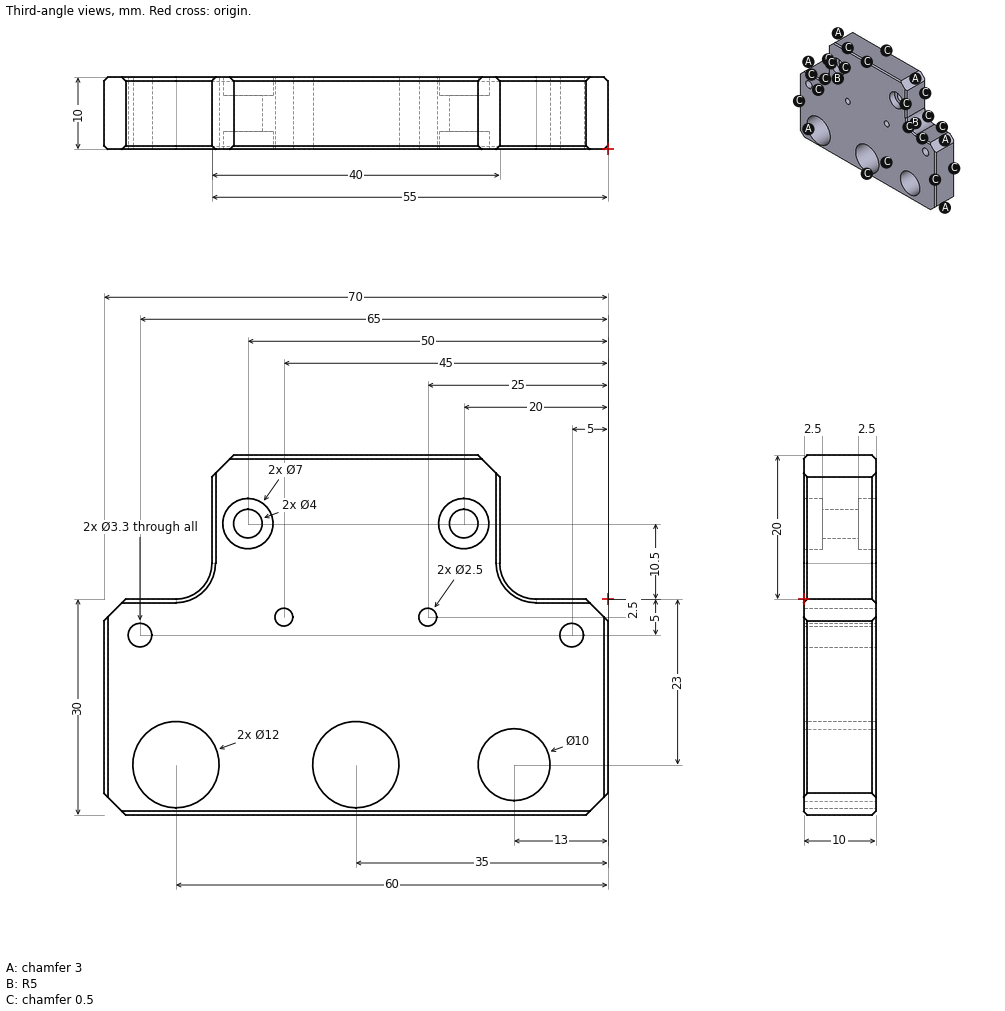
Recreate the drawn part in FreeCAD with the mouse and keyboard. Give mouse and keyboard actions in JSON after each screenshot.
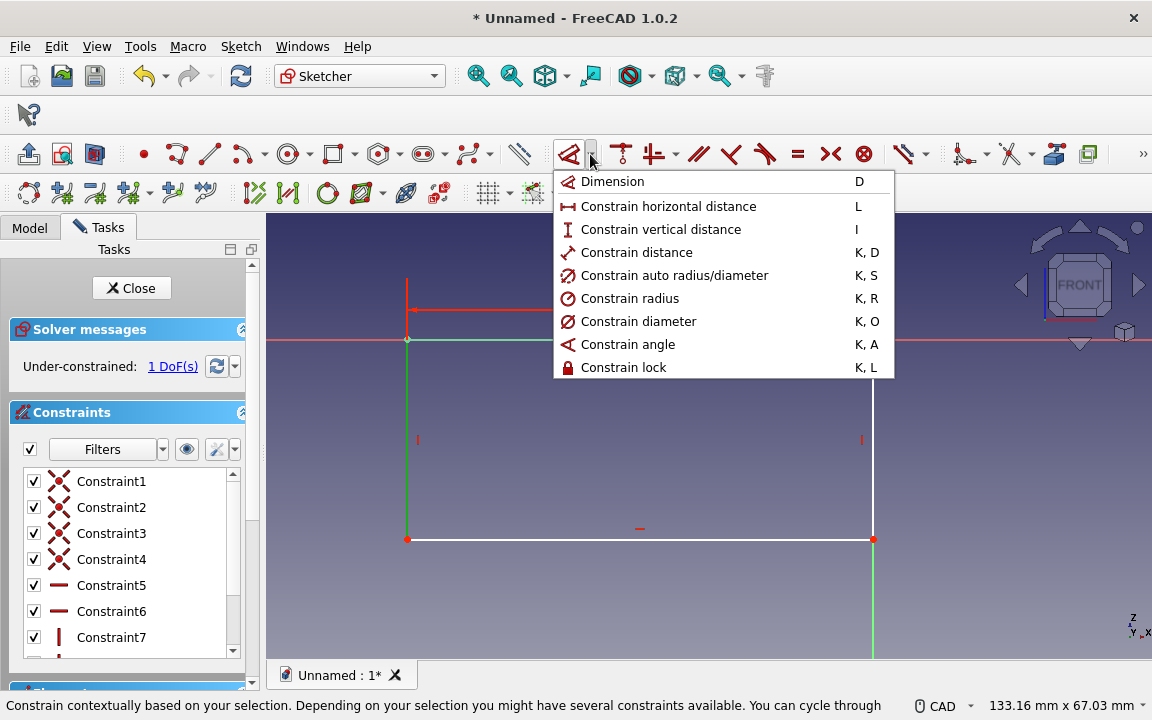
{"action": "left_click", "coordinate": [724, 230]}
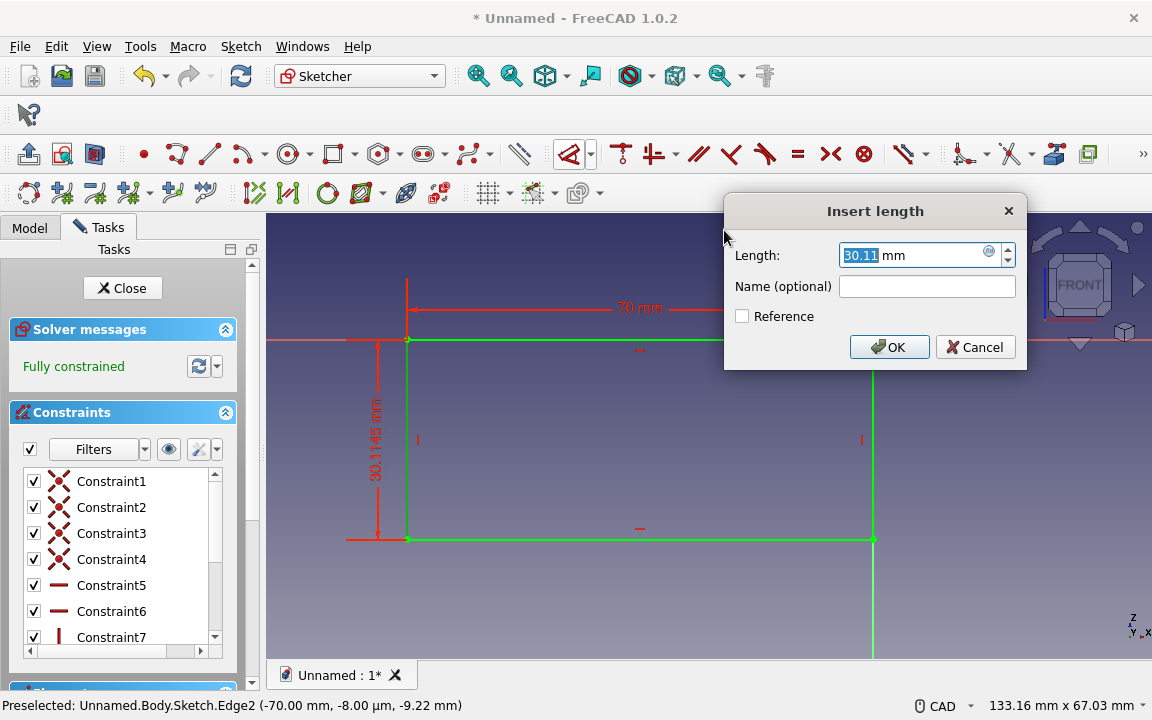
{"action": "type", "text": "30"}
{"action": "key", "text": "Return"}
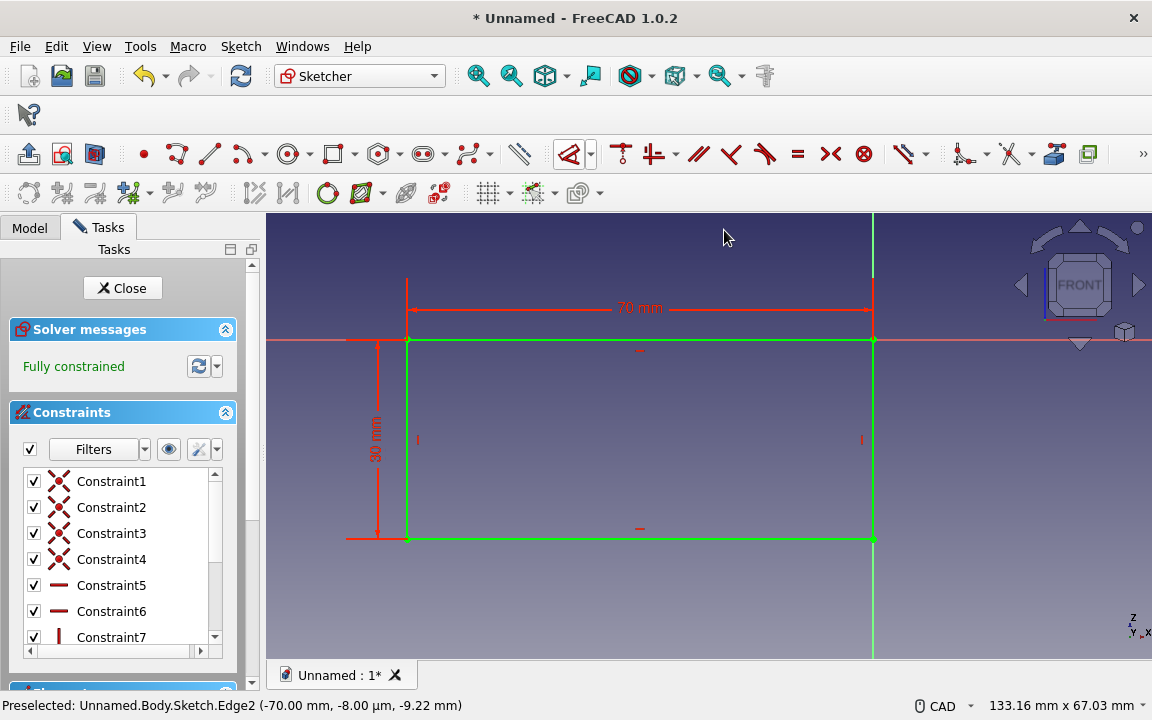
{"action": "left_click", "coordinate": [123, 288]}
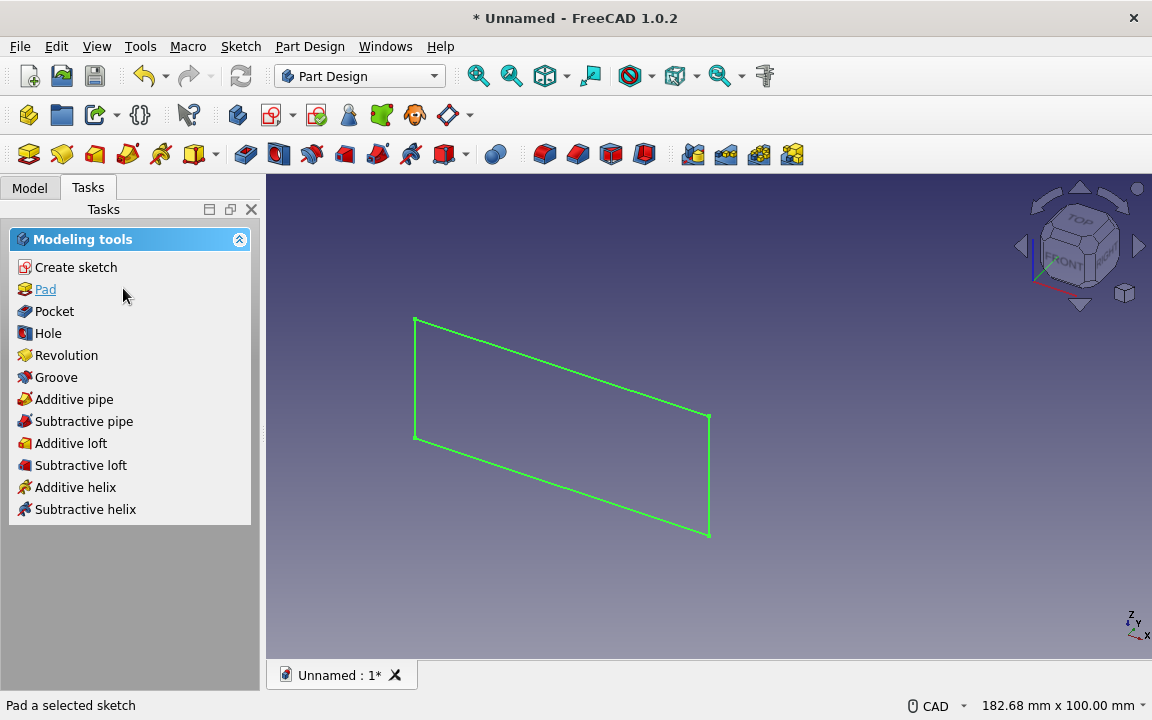
{"action": "left_click", "coordinate": [29, 154]}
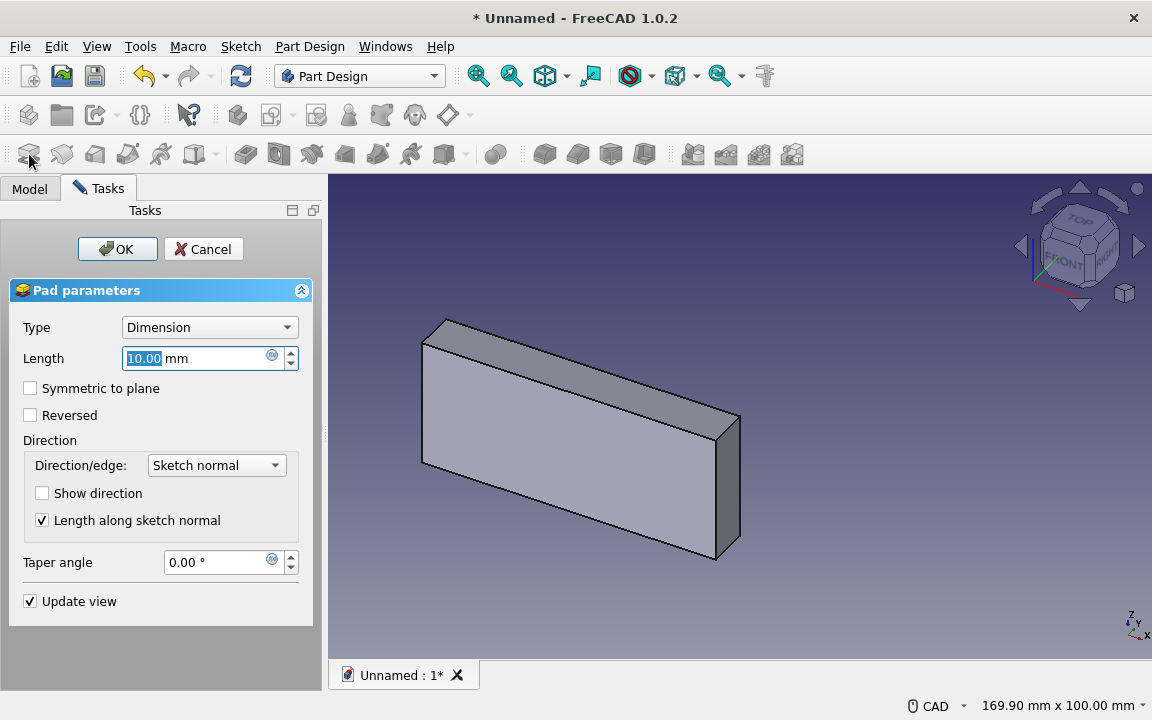
{"action": "type", "text": "10"}
{"action": "key", "text": "Tab"}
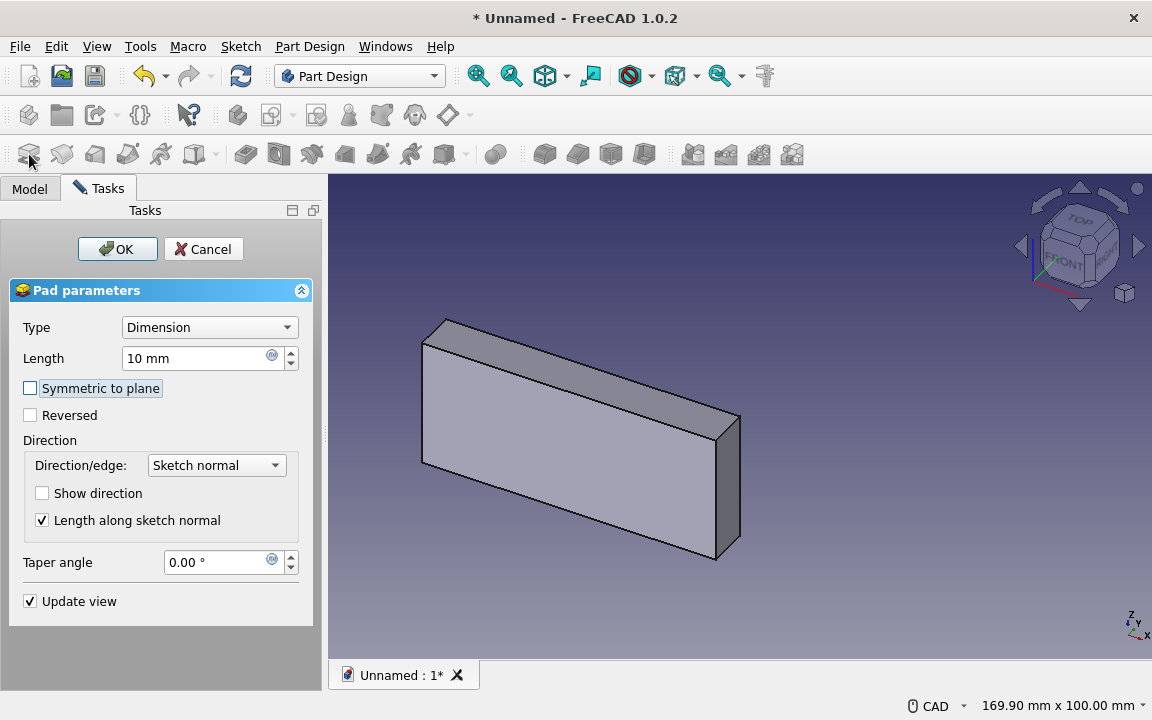
{"action": "left_click", "coordinate": [31, 415]}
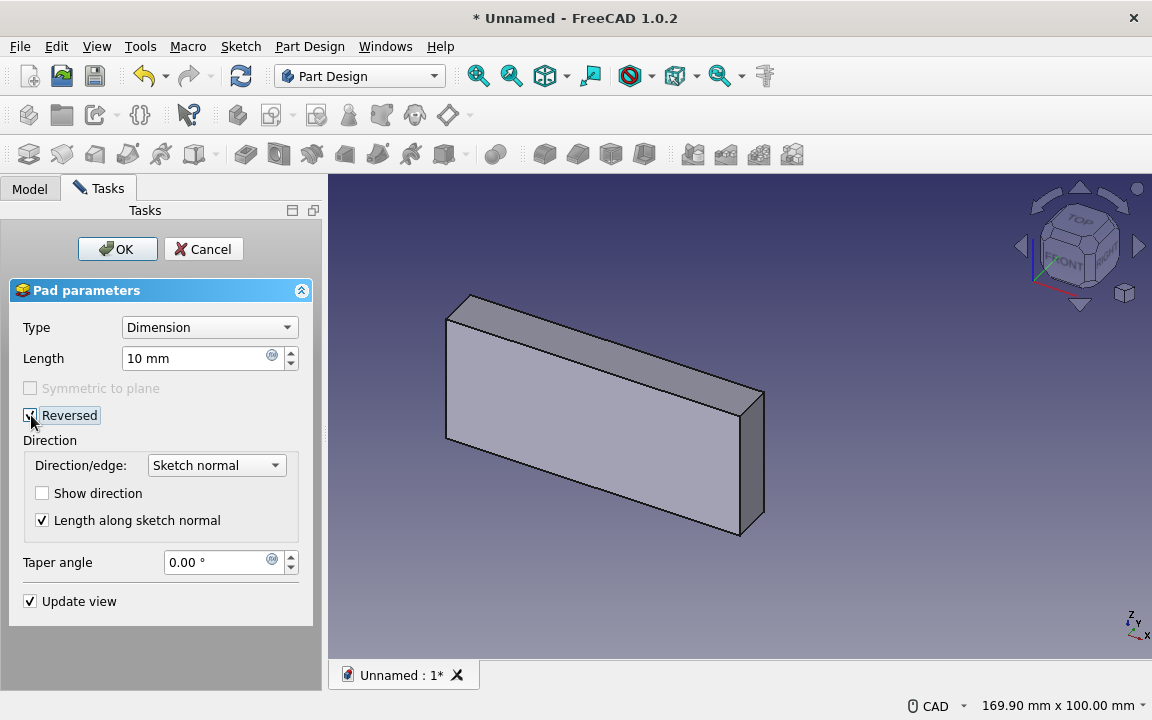
{"action": "left_click", "coordinate": [118, 249]}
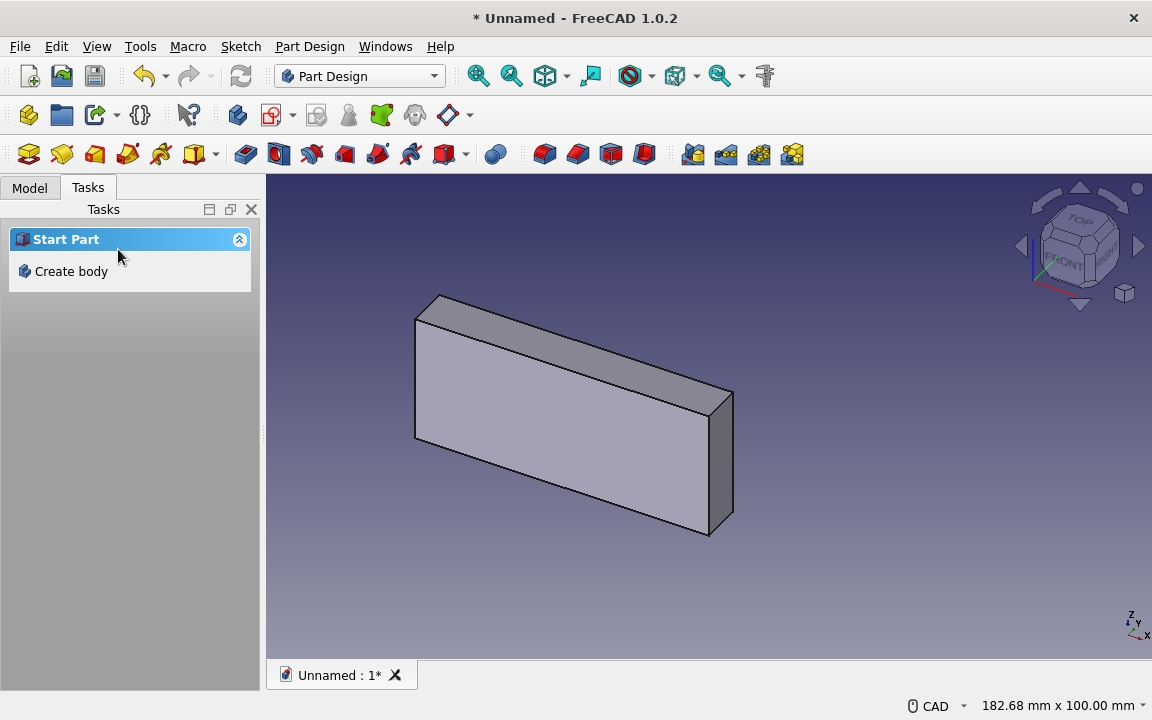
{"action": "left_click", "coordinate": [646, 454]}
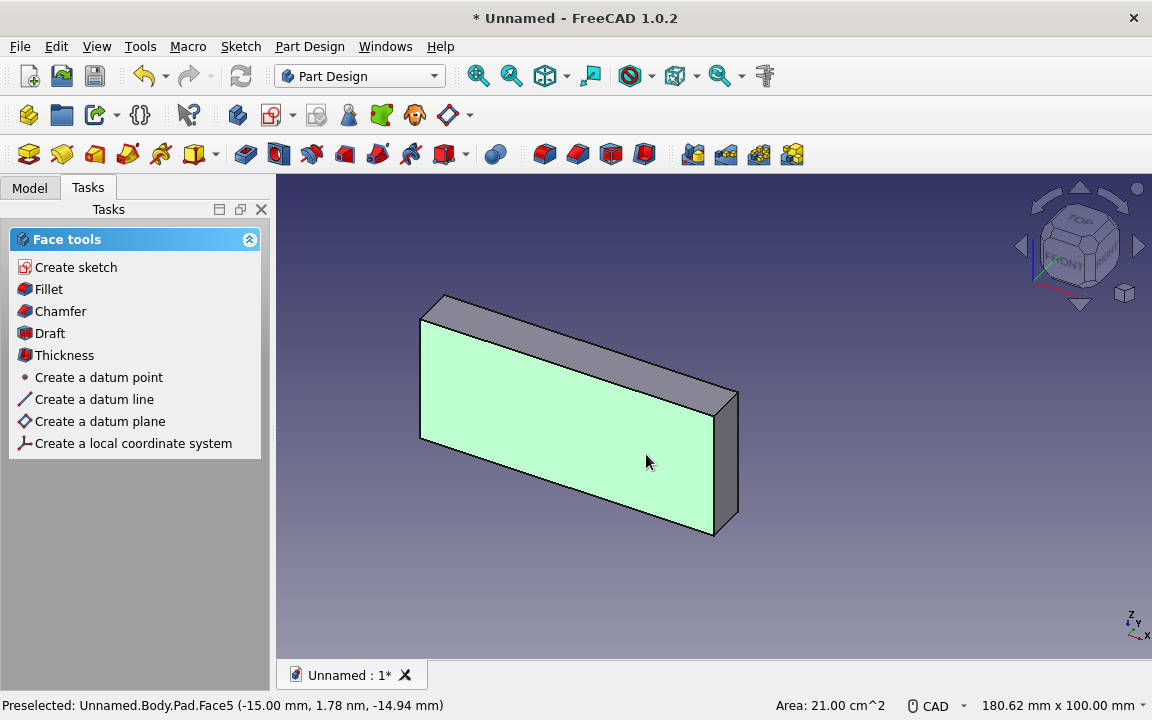
{"action": "left_click", "coordinate": [270, 116]}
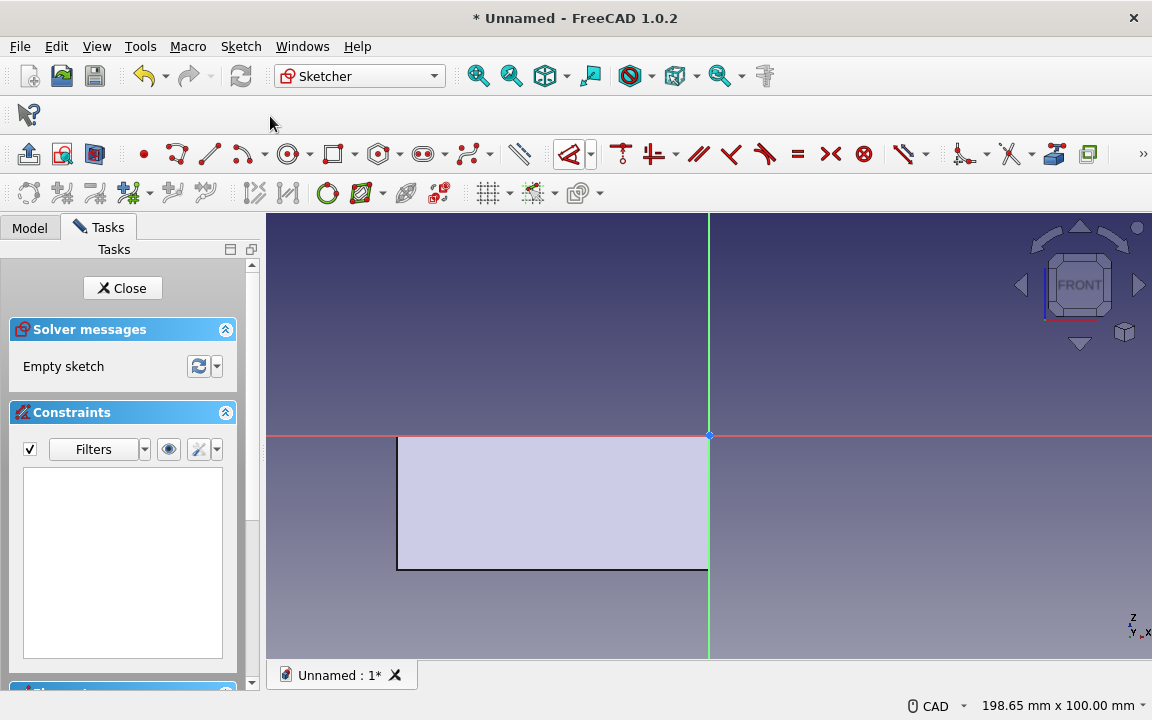
{"action": "scroll", "coordinate": [653, 559], "scroll_direction": "up", "scroll_amount": 9}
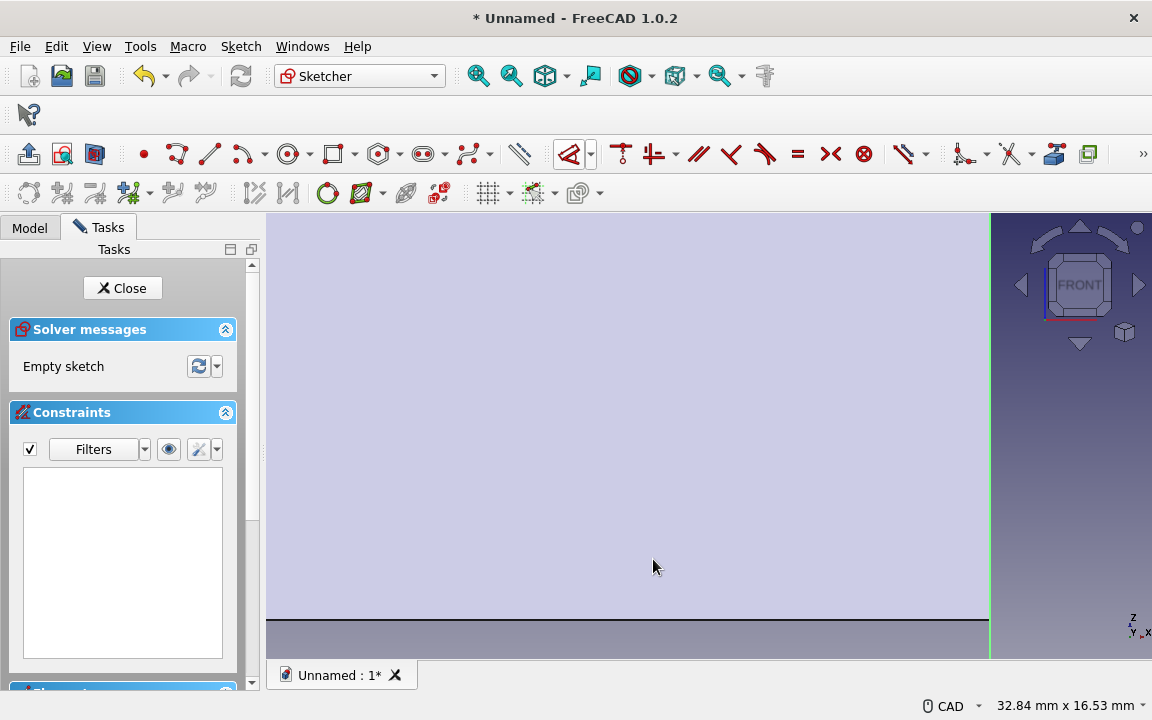
{"action": "left_click", "coordinate": [288, 154]}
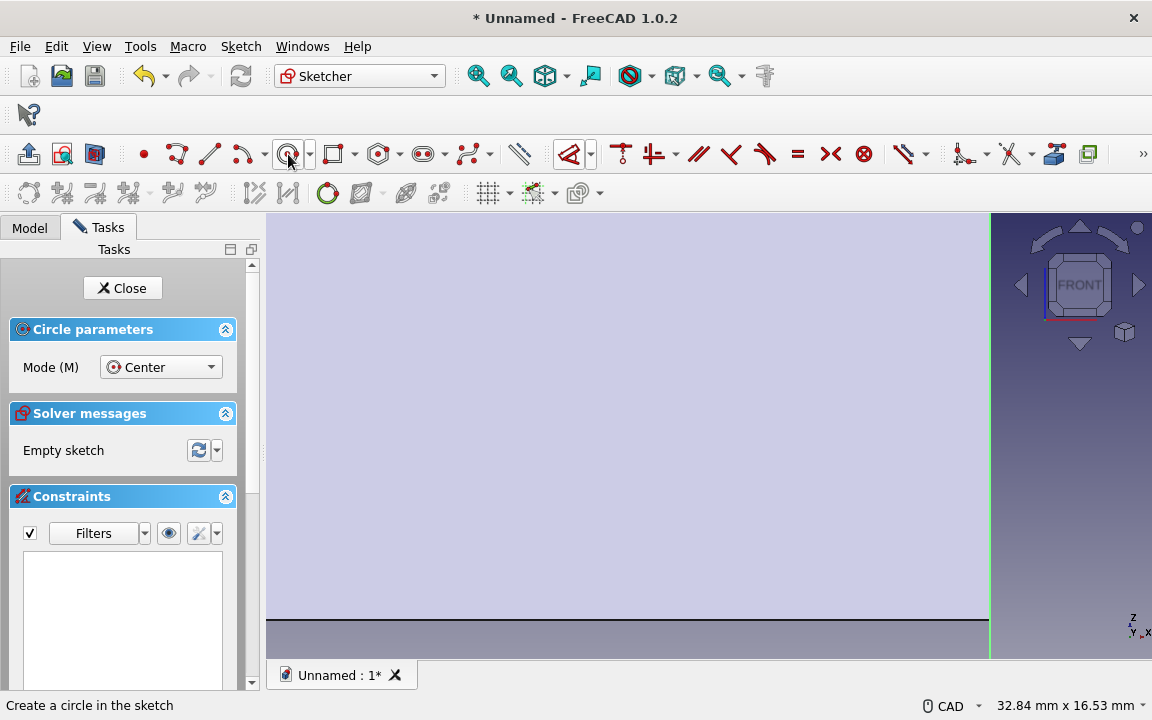
{"action": "left_click", "coordinate": [639, 432]}
{"action": "left_click", "coordinate": [734, 336]}
{"action": "key", "text": "Escape"}